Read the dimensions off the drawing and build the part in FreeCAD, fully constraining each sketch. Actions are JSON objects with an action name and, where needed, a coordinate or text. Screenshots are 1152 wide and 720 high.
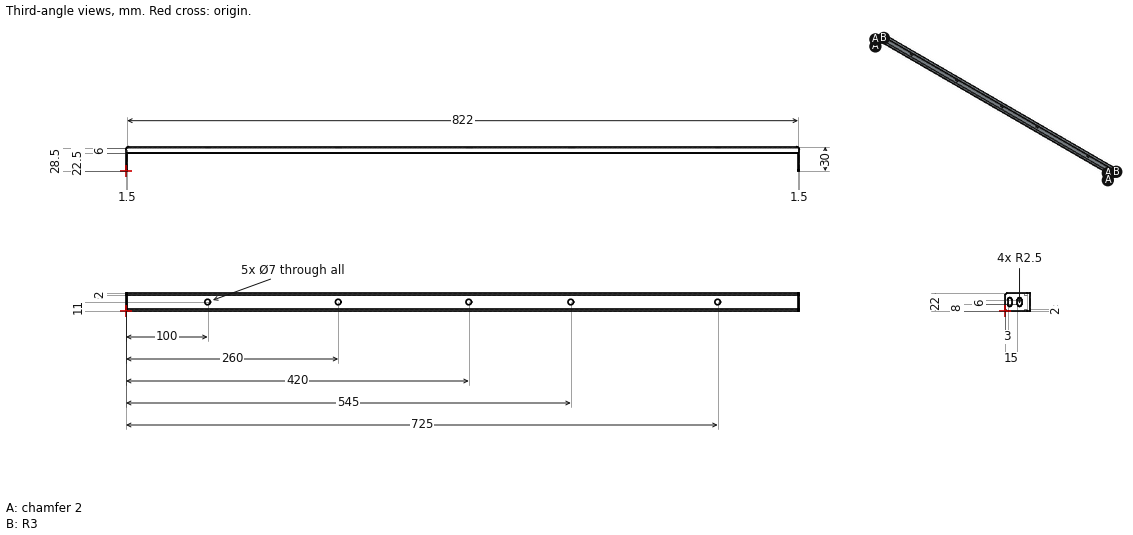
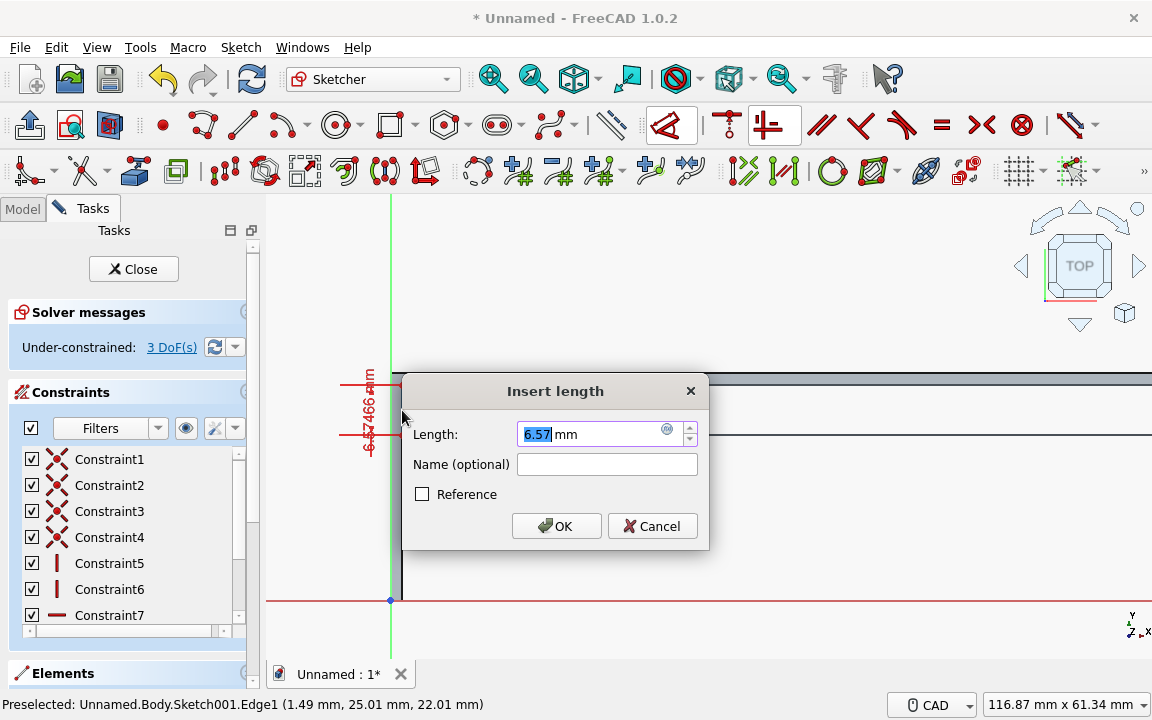
{"action": "type", "text": "6"}
{"action": "key", "text": "Return"}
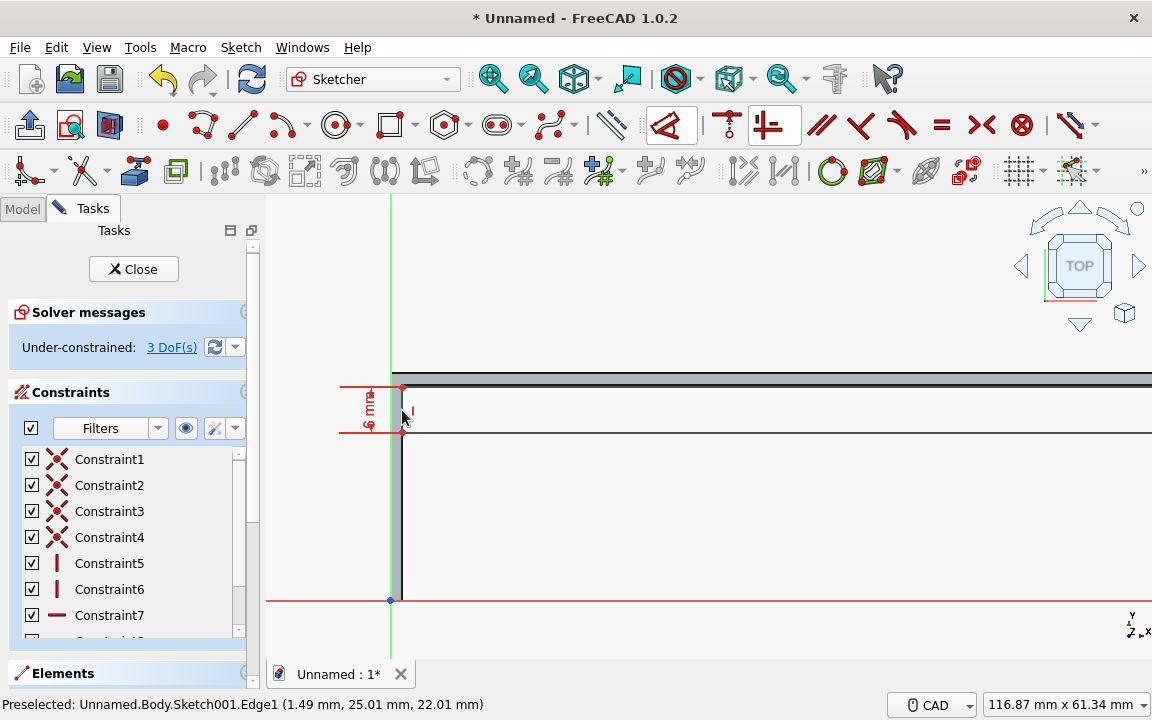
{"action": "scroll", "coordinate": [410, 421], "scroll_direction": "down", "scroll_amount": 13}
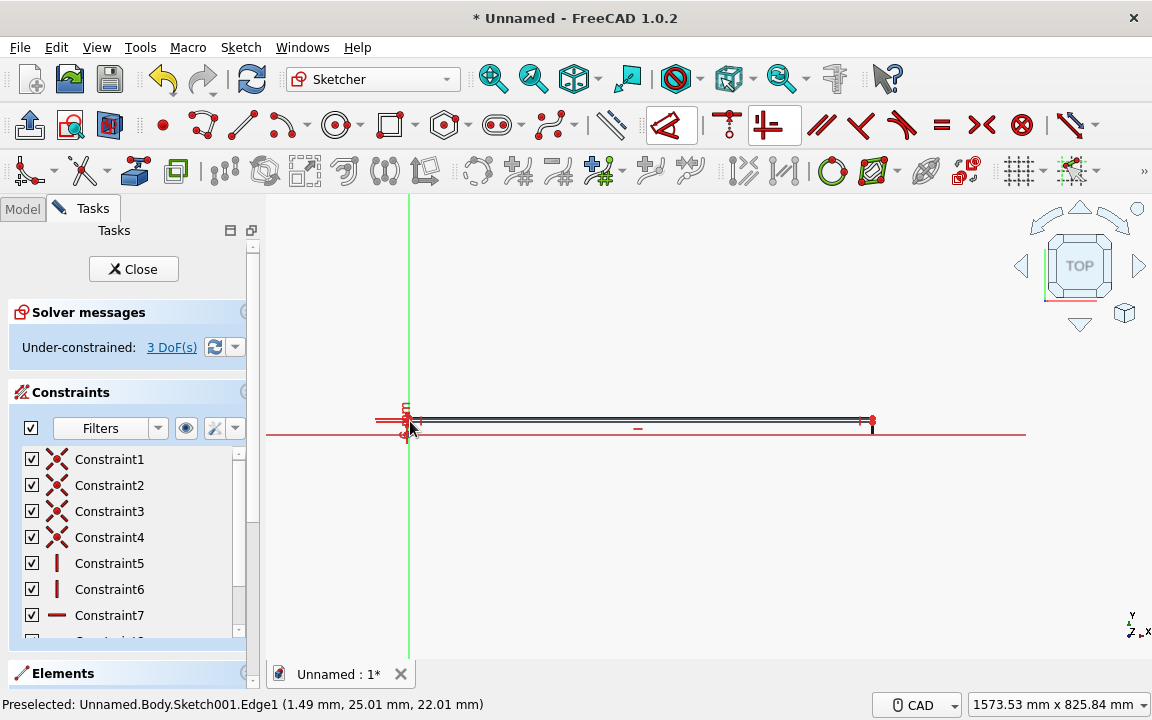
{"action": "scroll", "coordinate": [548, 422], "scroll_direction": "up", "scroll_amount": 8}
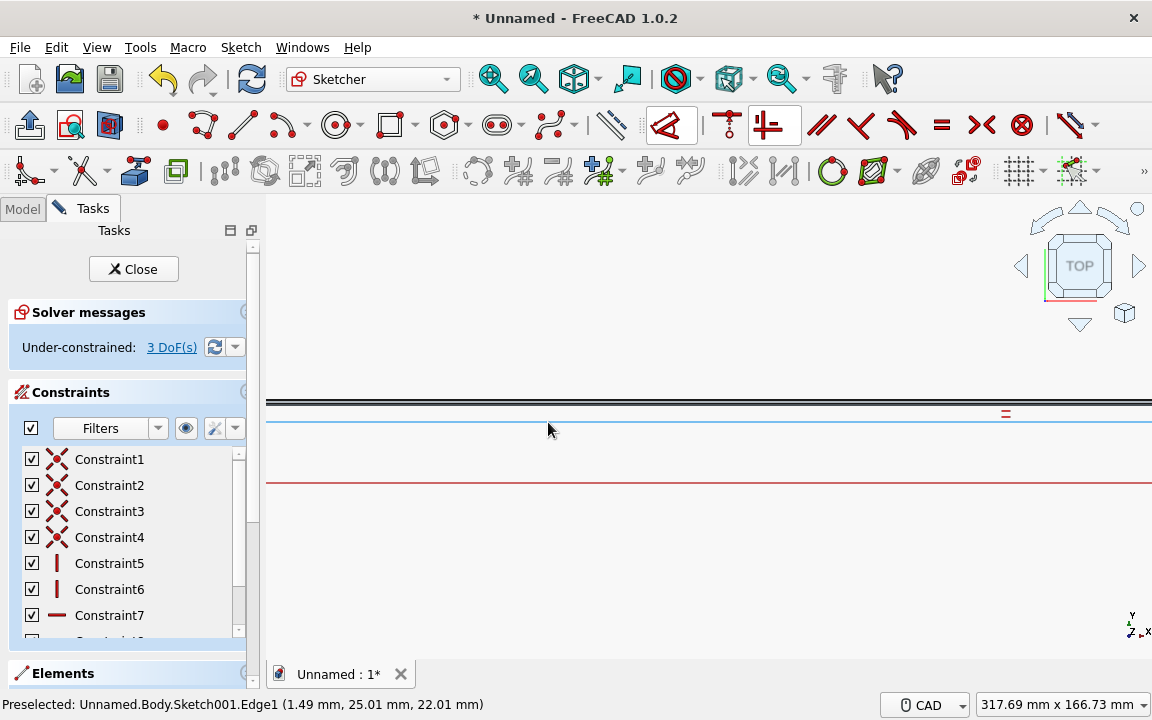
{"action": "left_click", "coordinate": [549, 422]}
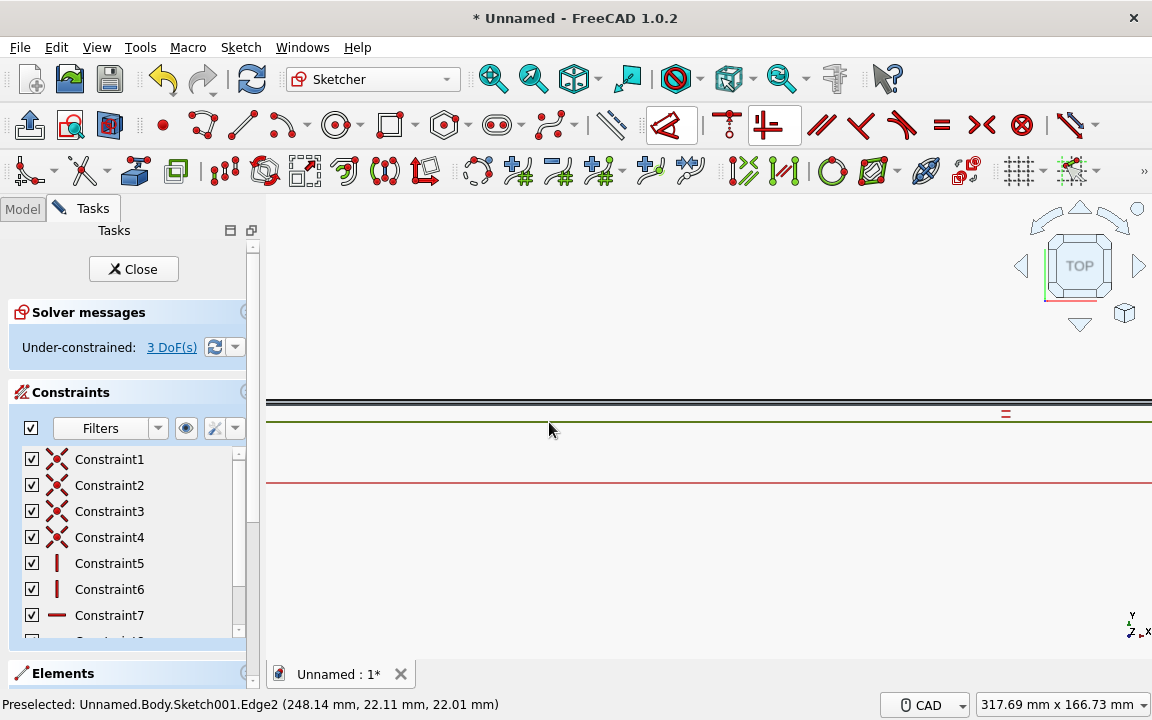
{"action": "key", "text": "l"}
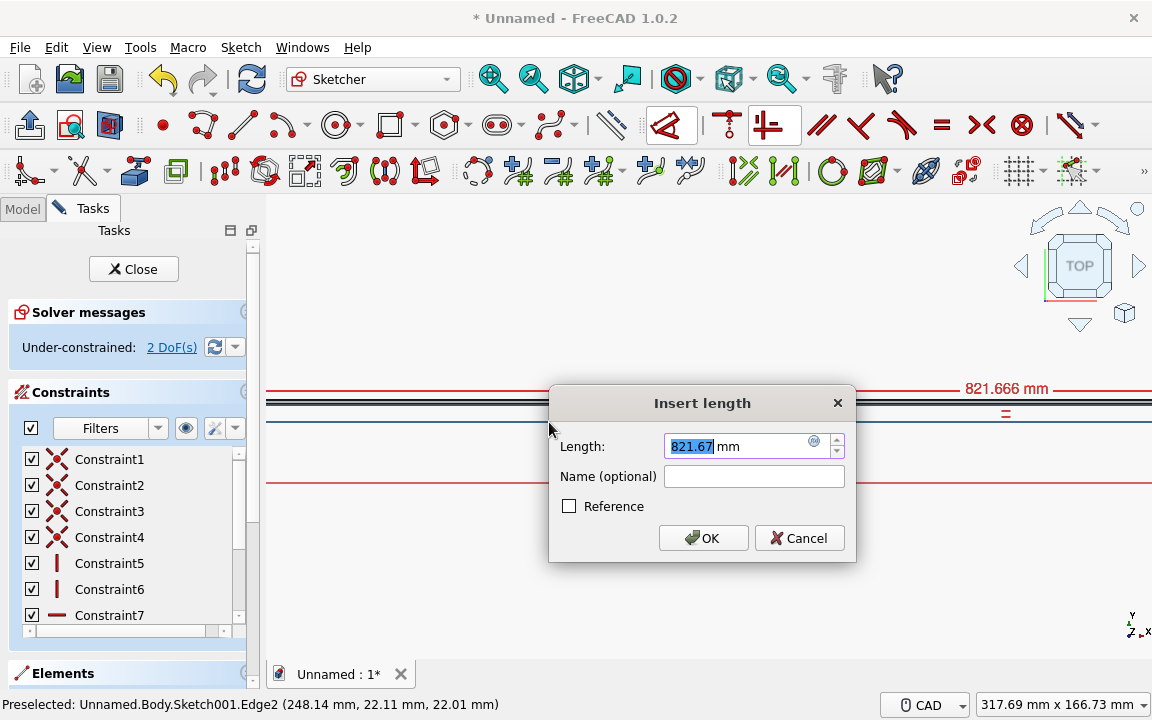
{"action": "type", "text": "822"}
{"action": "key", "text": "Return"}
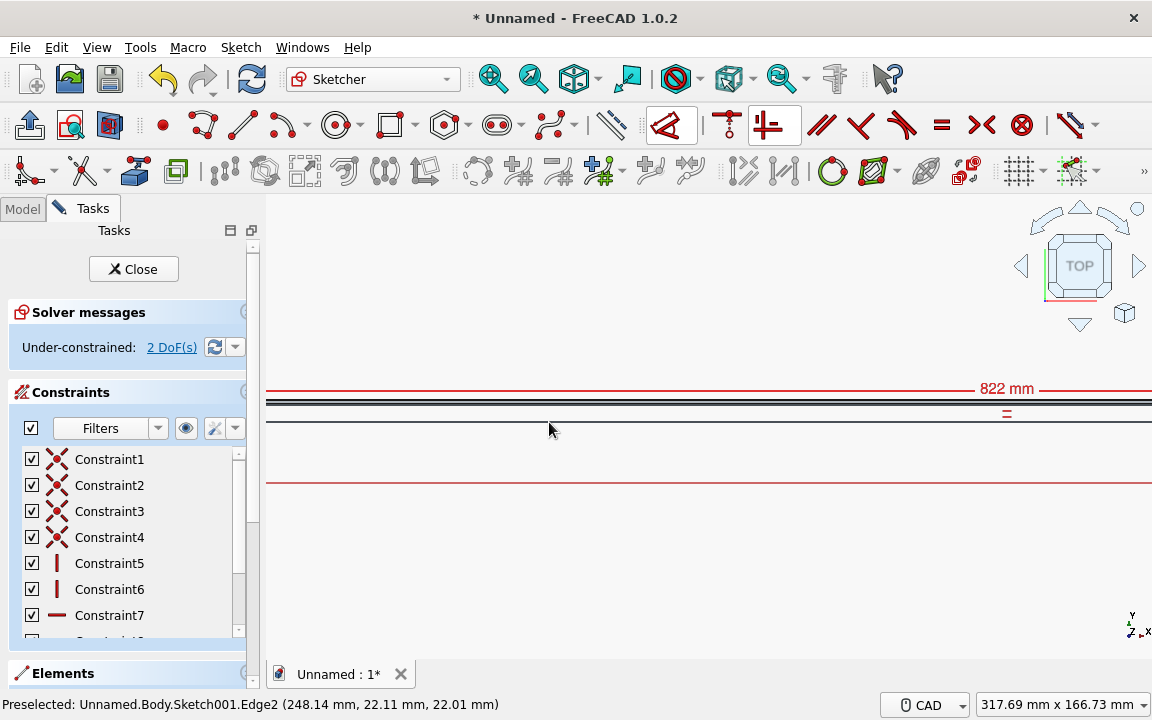
{"action": "scroll", "coordinate": [548, 422], "scroll_direction": "down", "scroll_amount": 8}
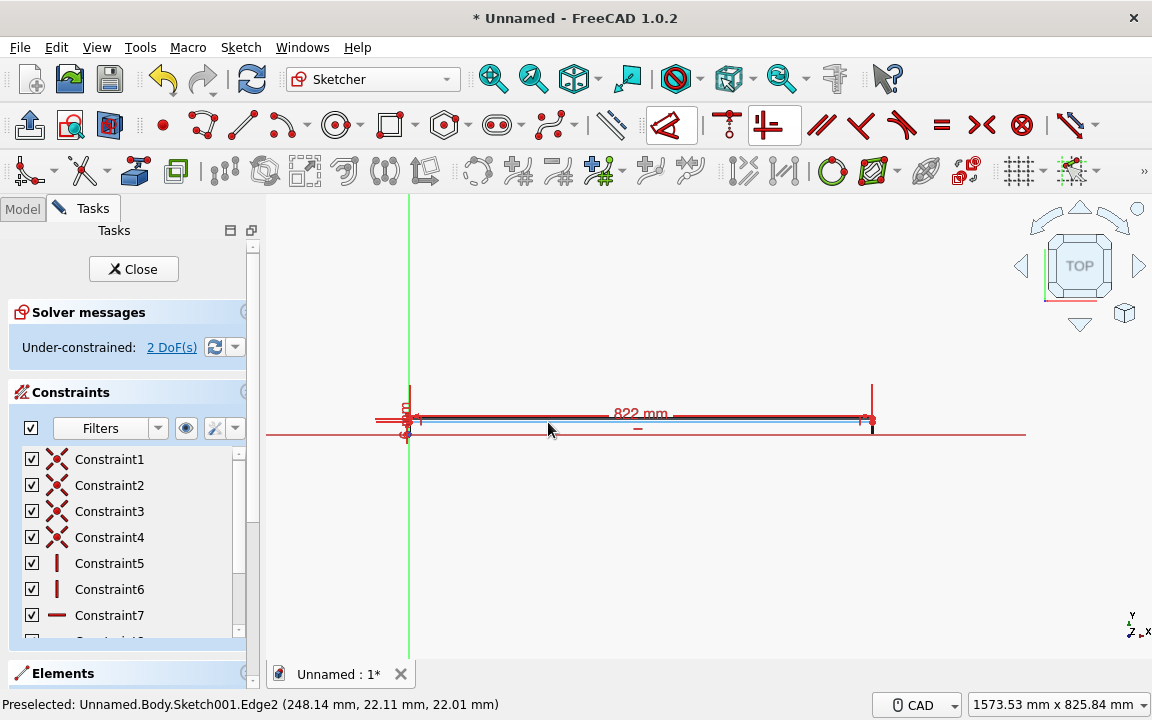
{"action": "scroll", "coordinate": [410, 419], "scroll_direction": "up", "scroll_amount": 20}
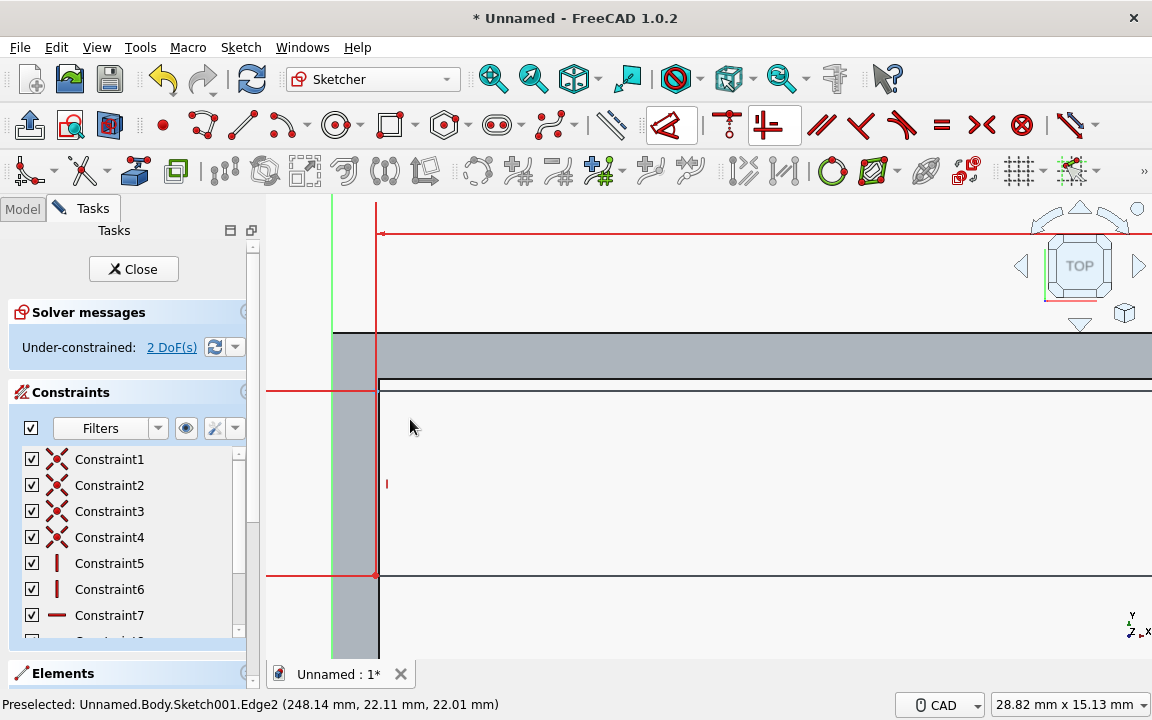
{"action": "left_click", "coordinate": [376, 391]}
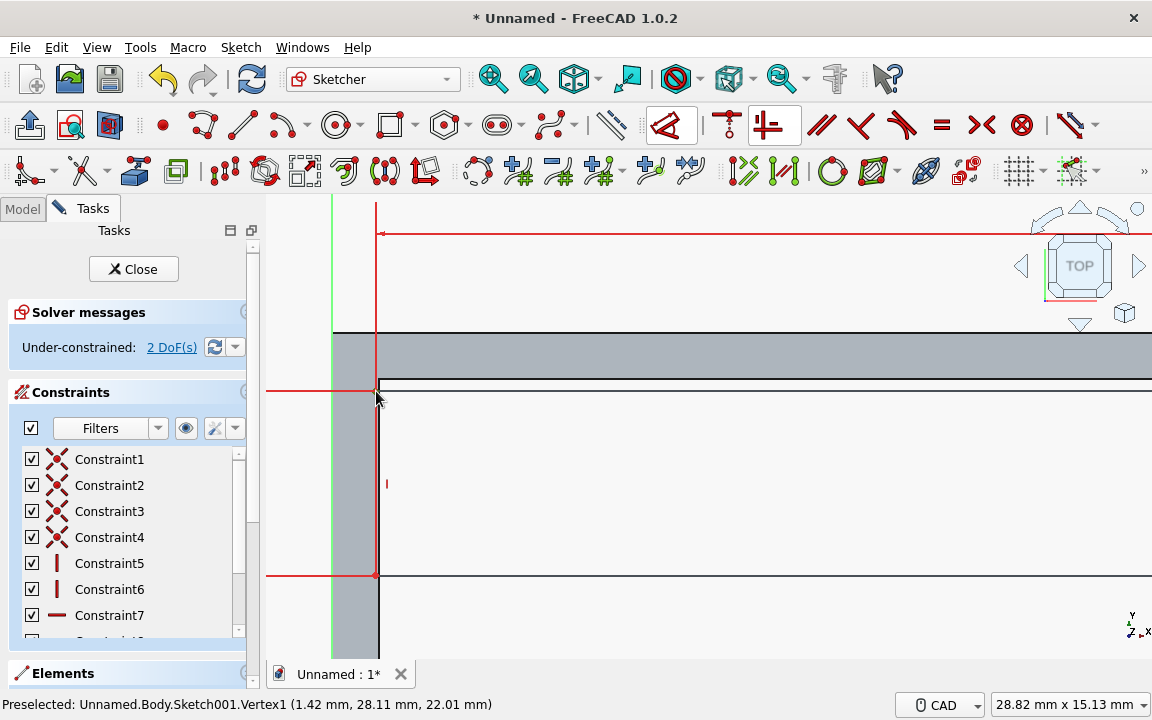
{"action": "left_click", "coordinate": [692, 126]}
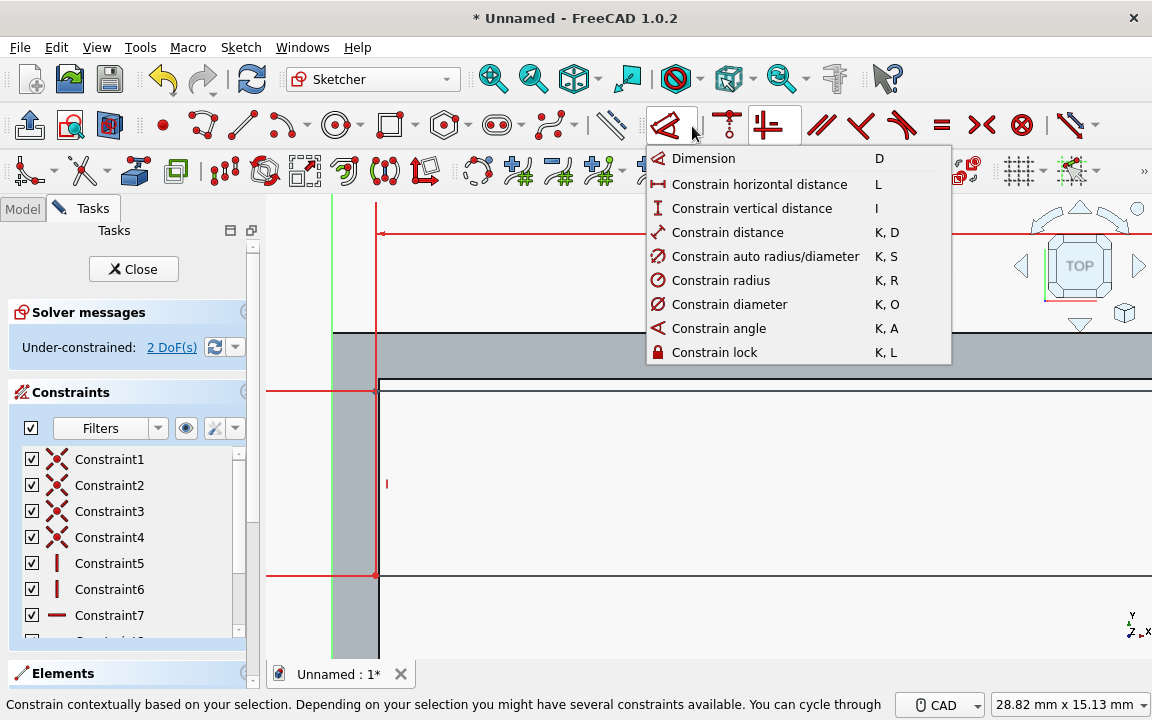
{"action": "left_click", "coordinate": [799, 184]}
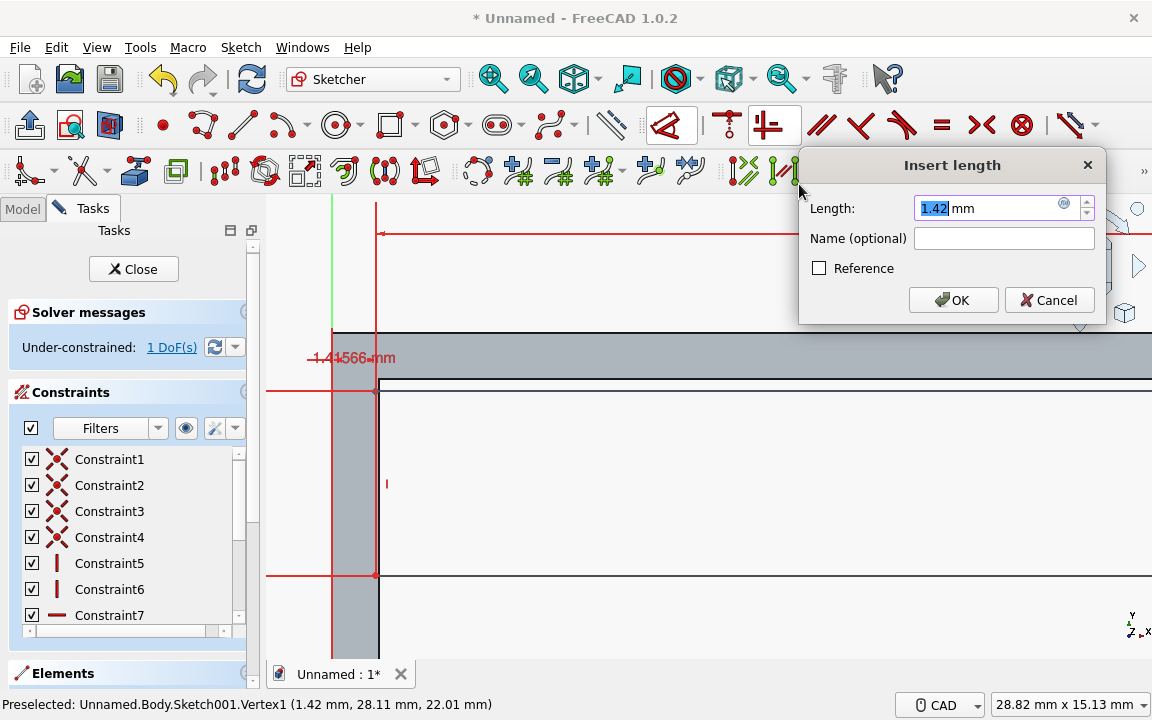
{"action": "type", "text": "1.5"}
{"action": "key", "text": "Return"}